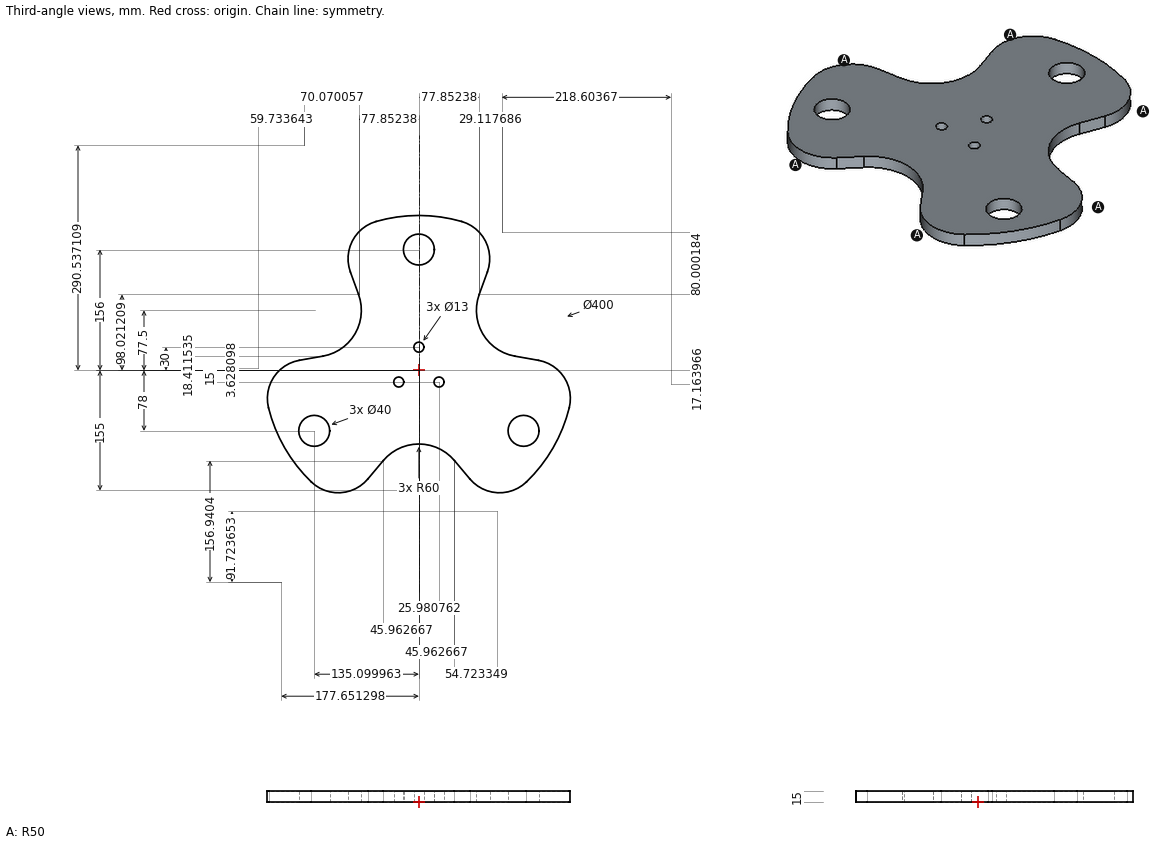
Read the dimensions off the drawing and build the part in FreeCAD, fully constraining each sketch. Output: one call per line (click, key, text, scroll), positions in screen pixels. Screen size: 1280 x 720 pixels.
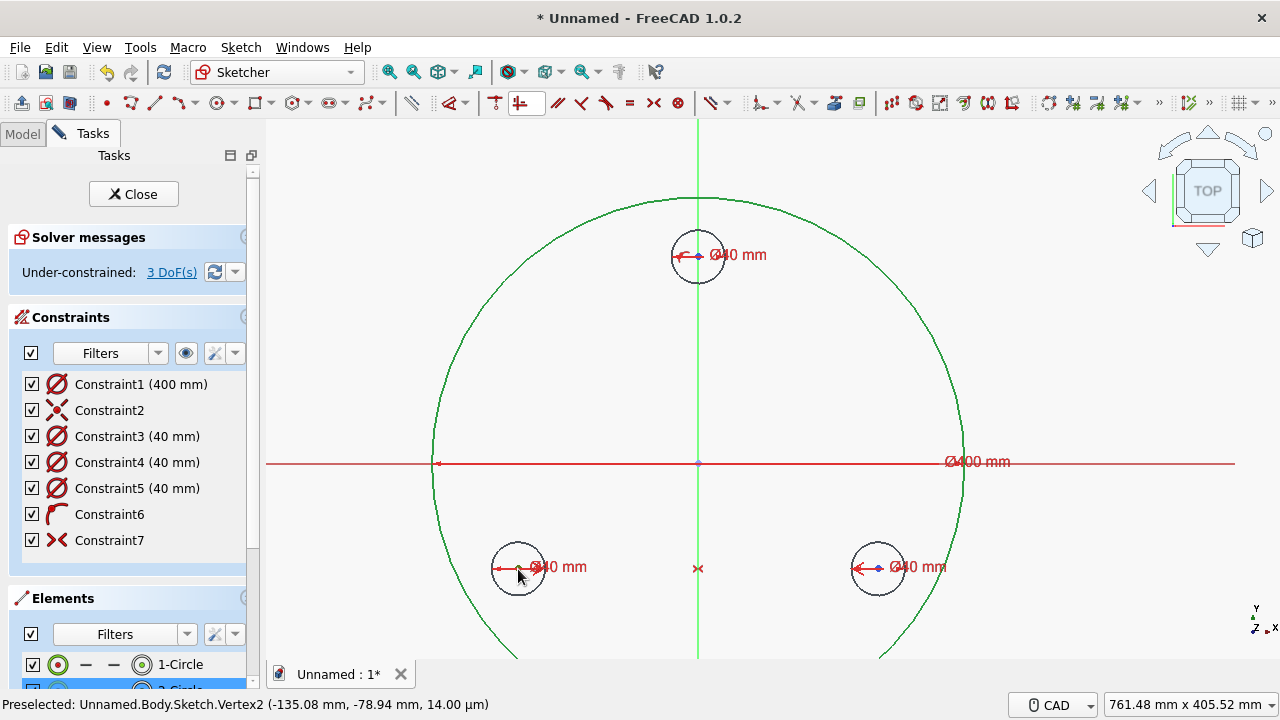
key(i)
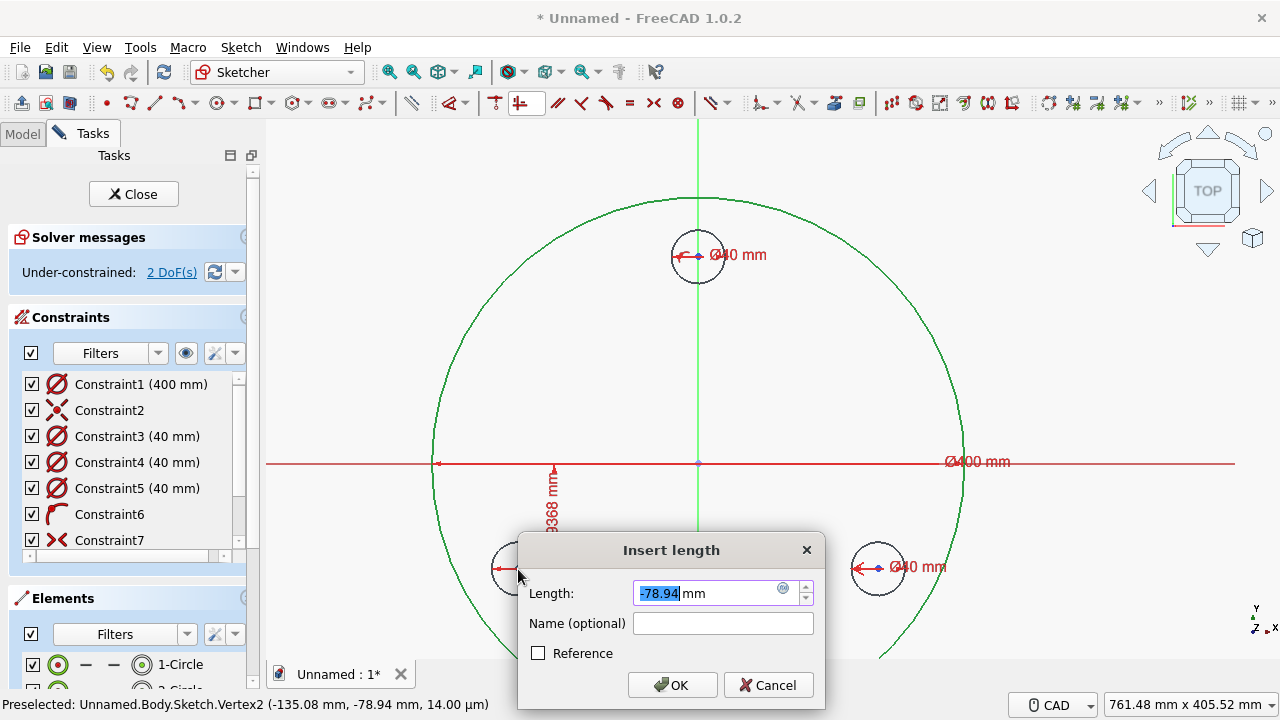
text(-78)
key(Return)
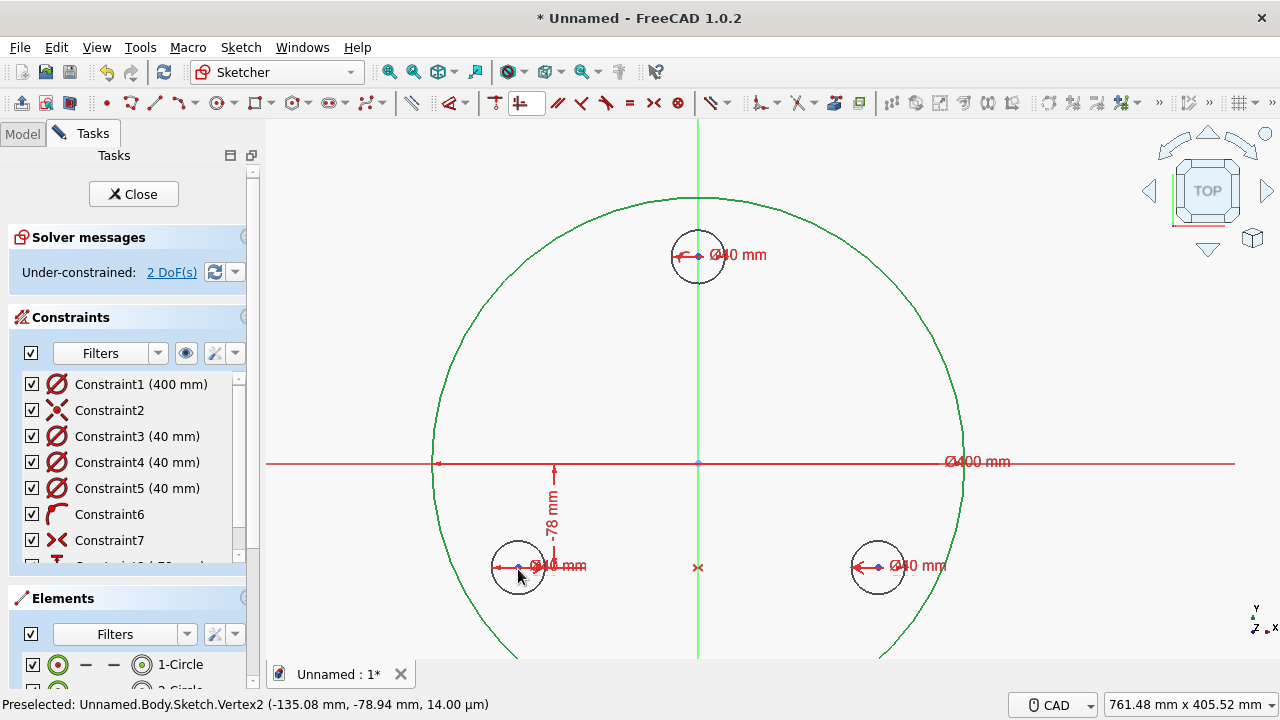
click(698, 257)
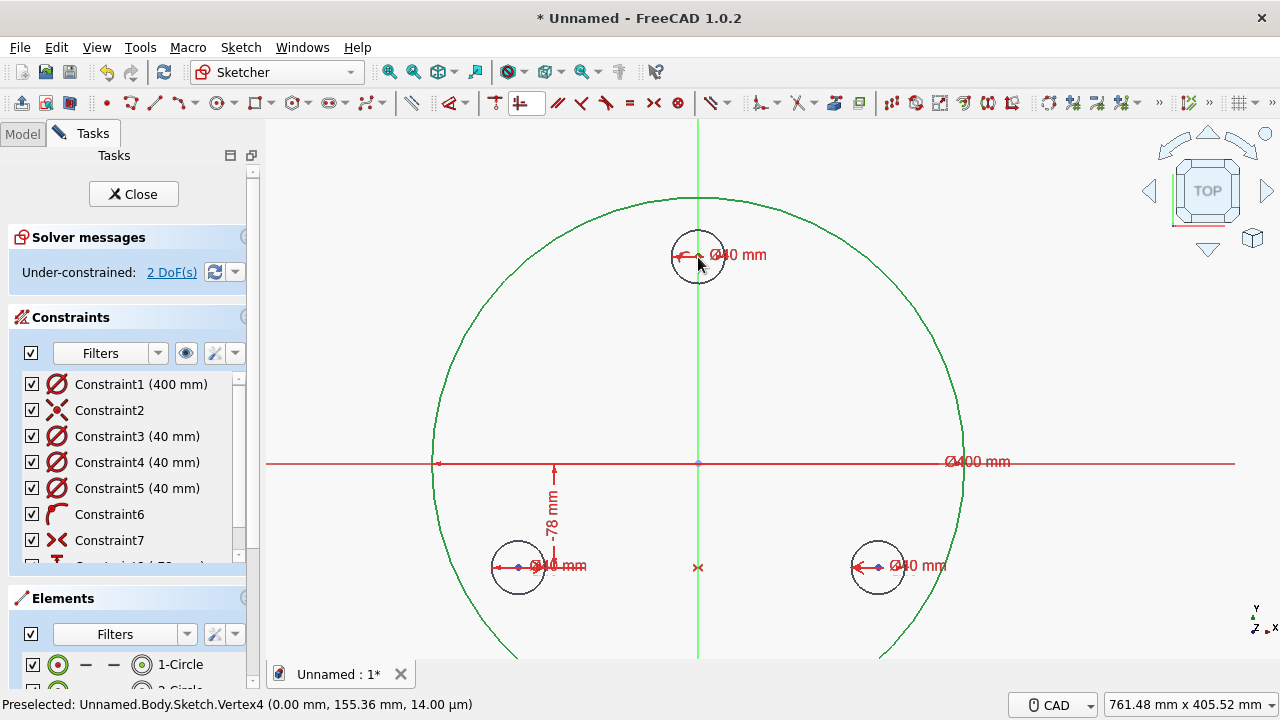
click(468, 104)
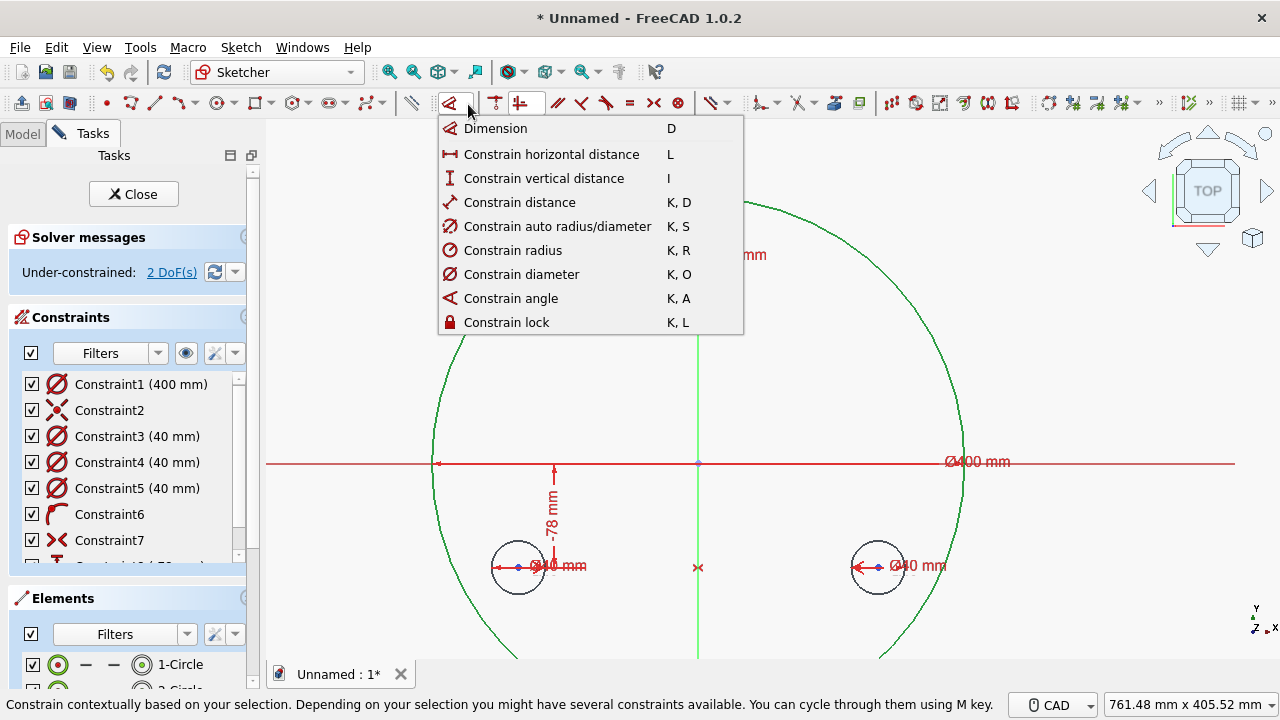
click(591, 178)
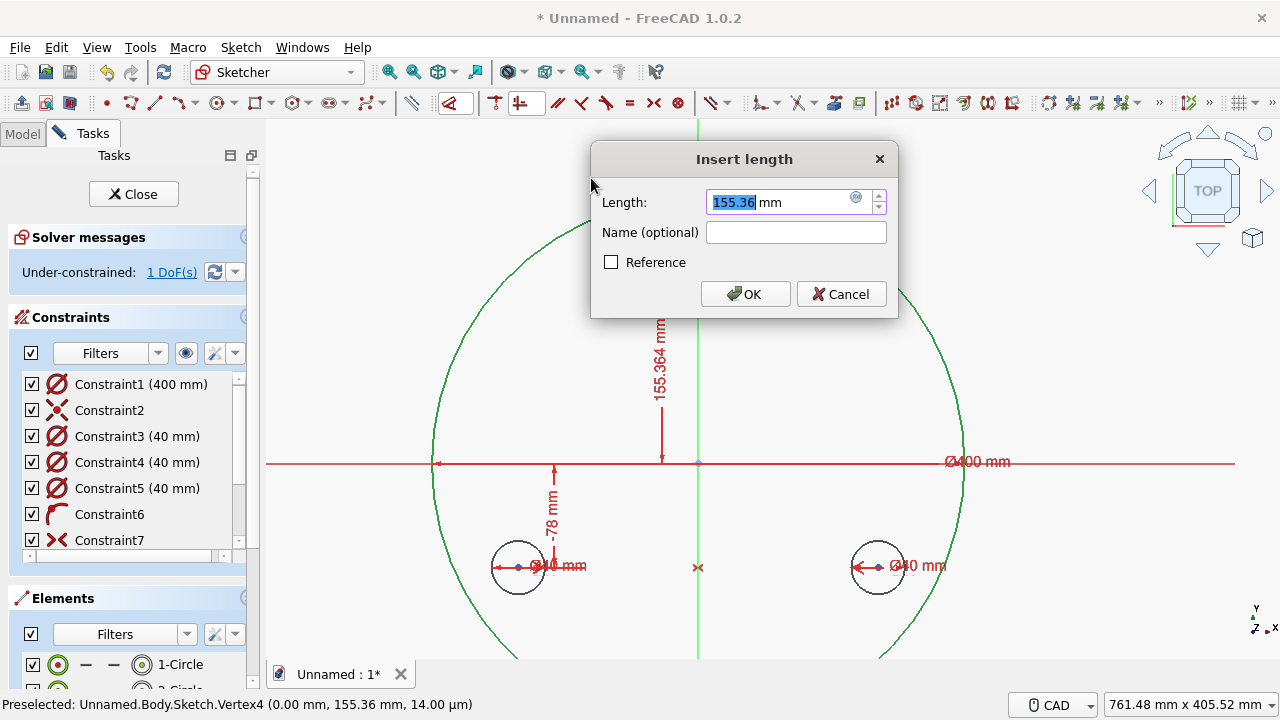
text(156)
key(Return)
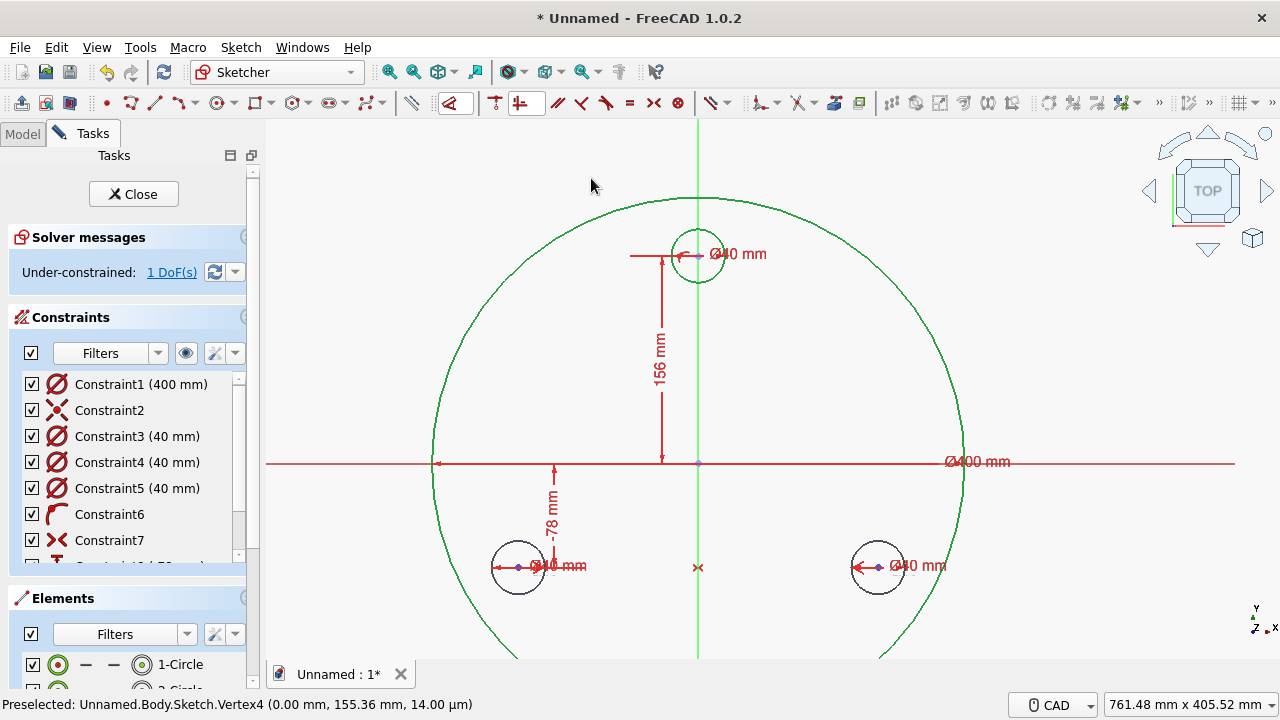
click(518, 568)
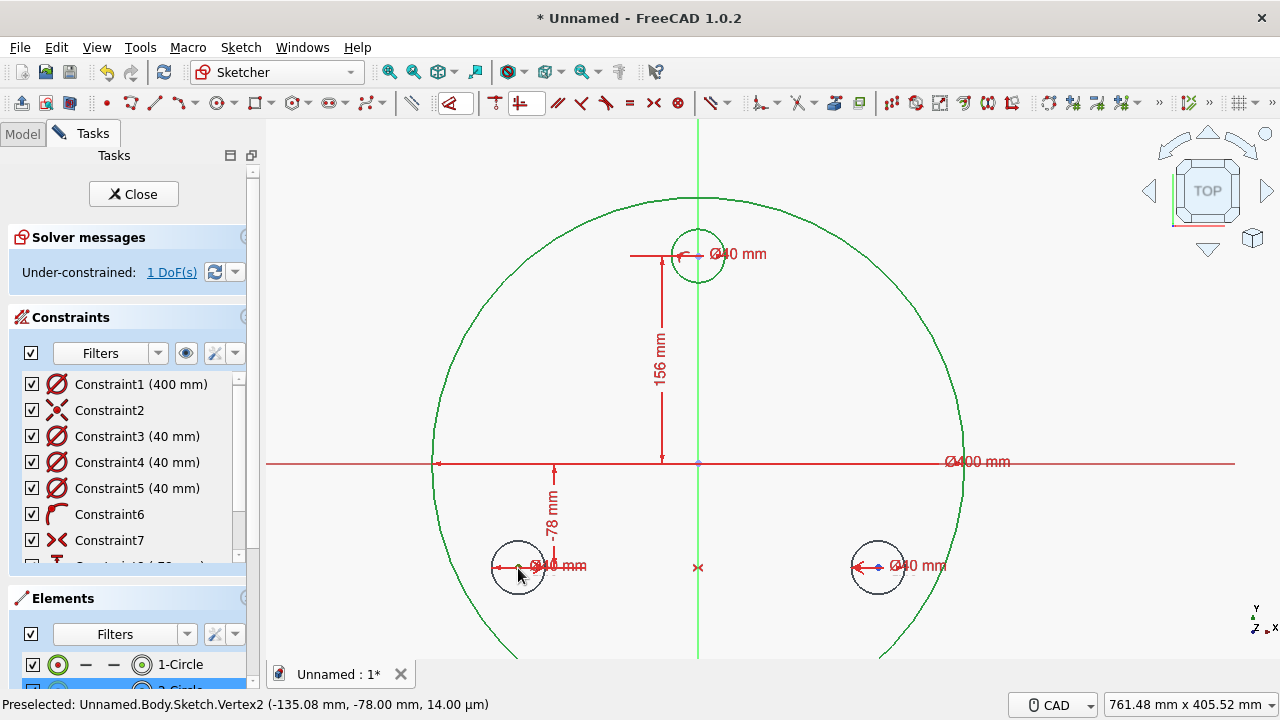
key(l)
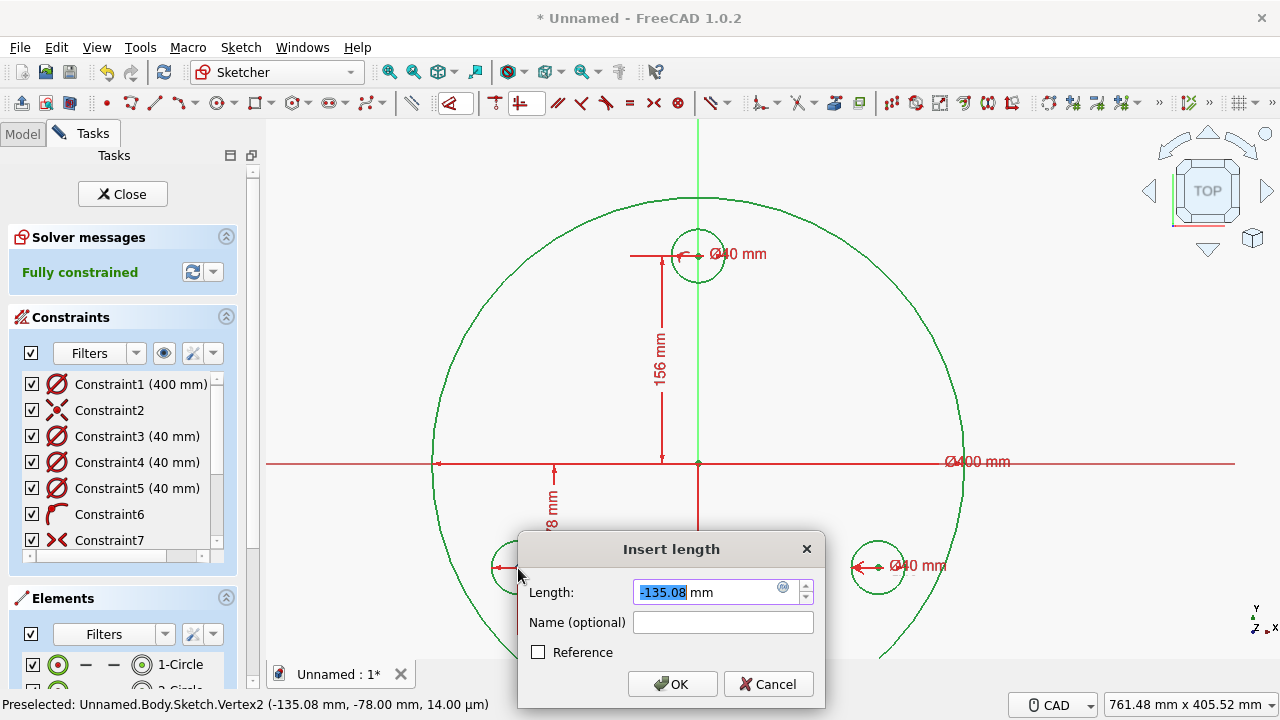
text(-135.099963)
key(Return)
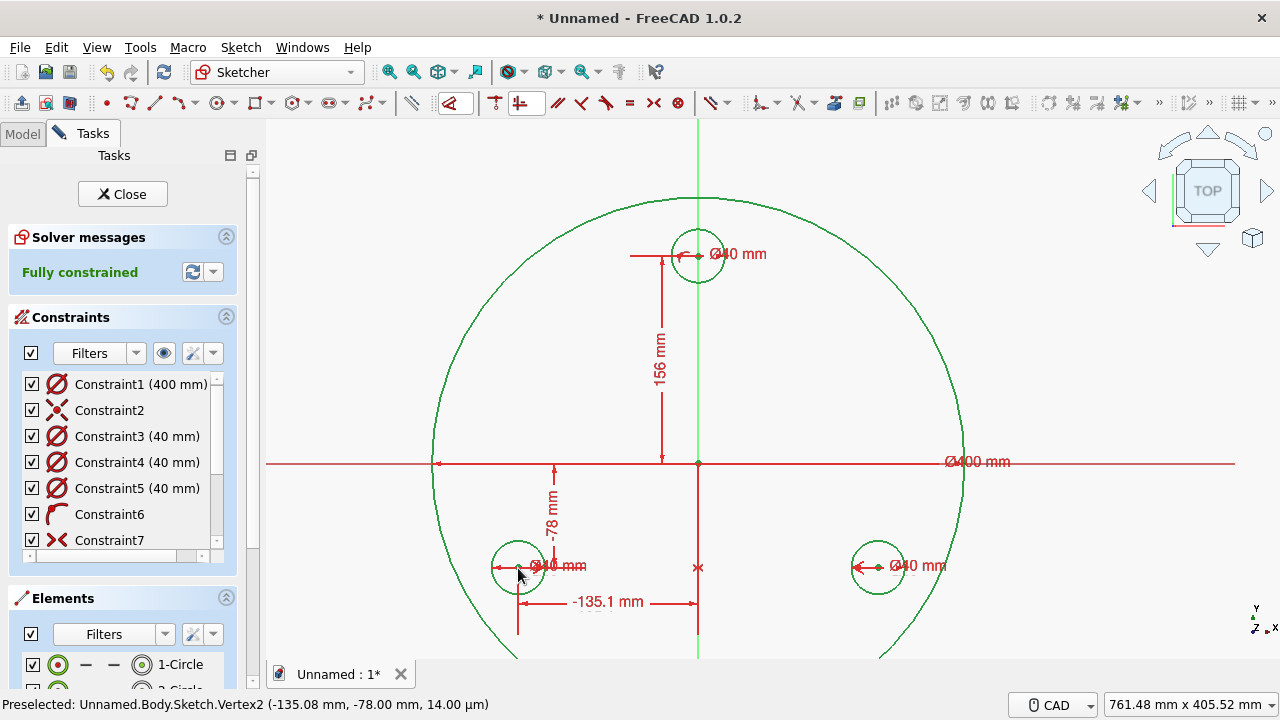
click(123, 194)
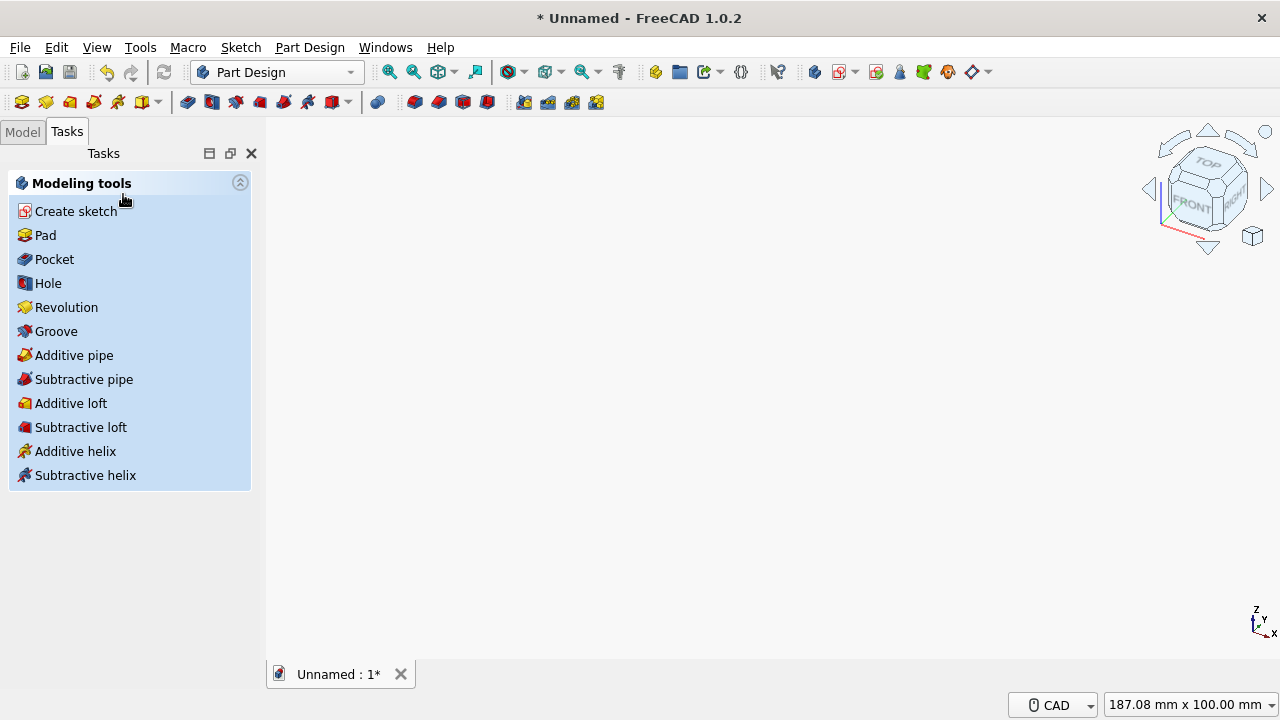
click(22, 102)